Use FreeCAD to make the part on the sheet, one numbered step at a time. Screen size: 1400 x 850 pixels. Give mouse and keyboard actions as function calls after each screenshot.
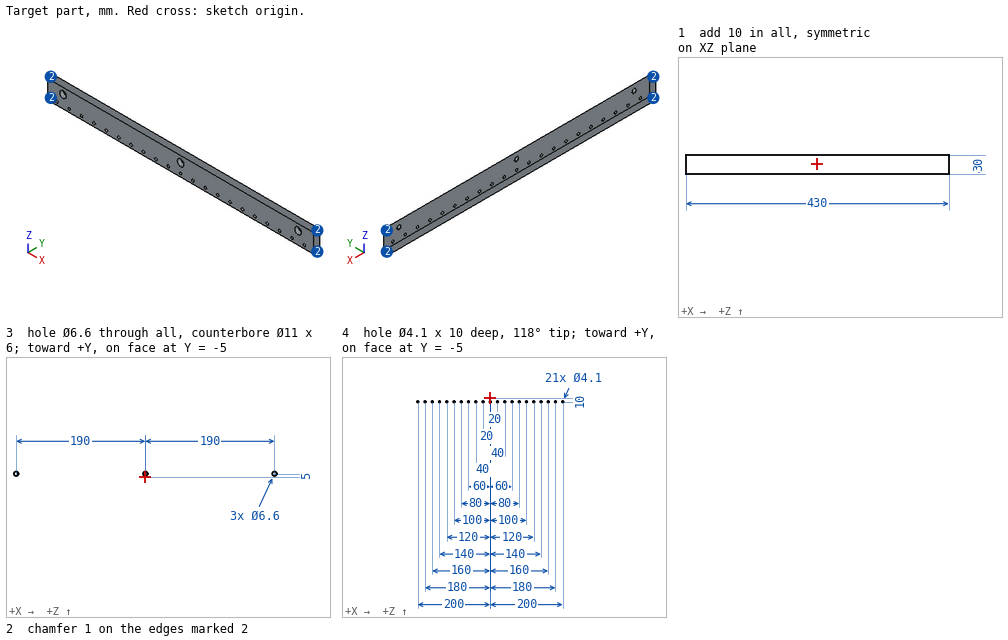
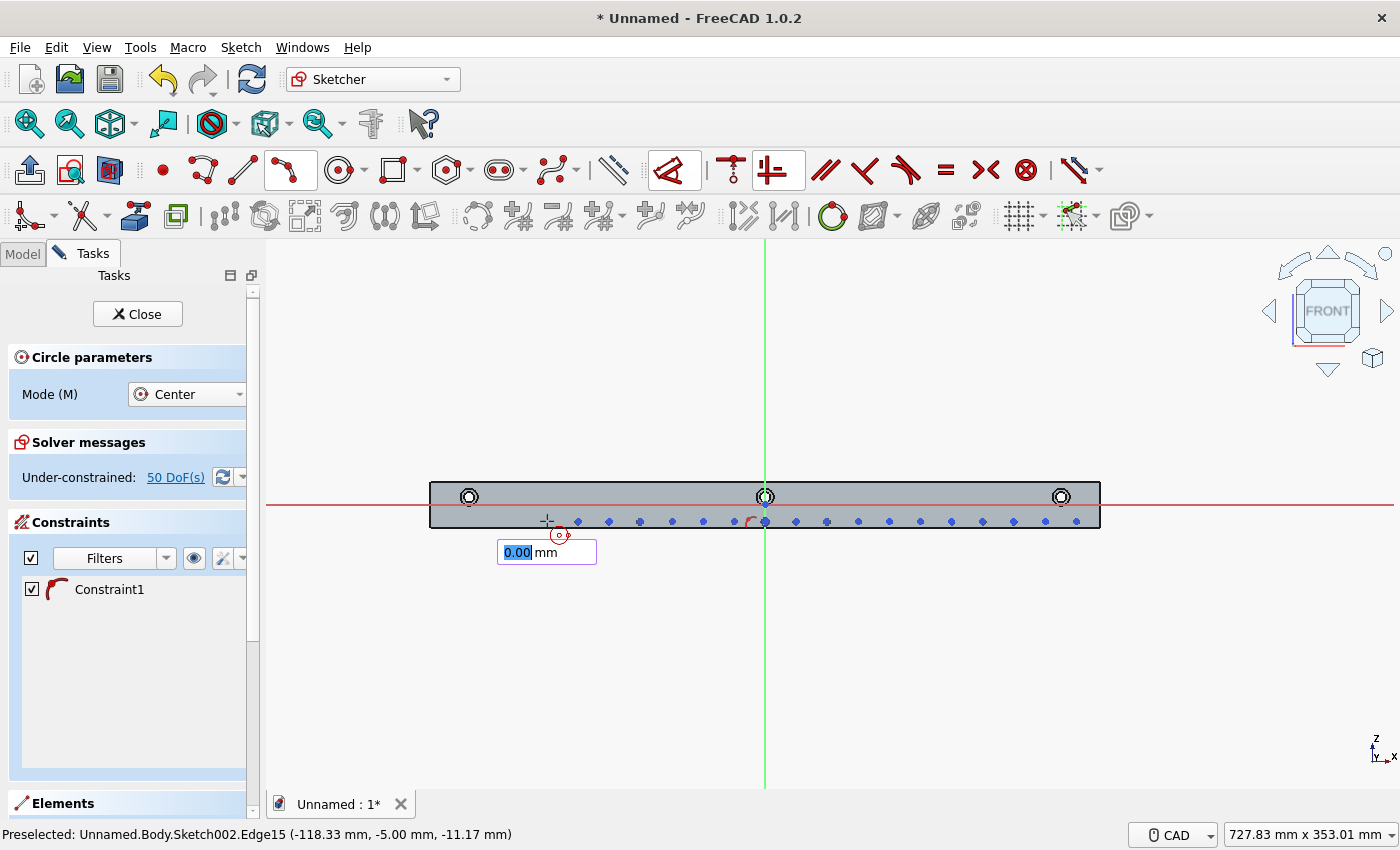
scroll(549, 523, up, 9)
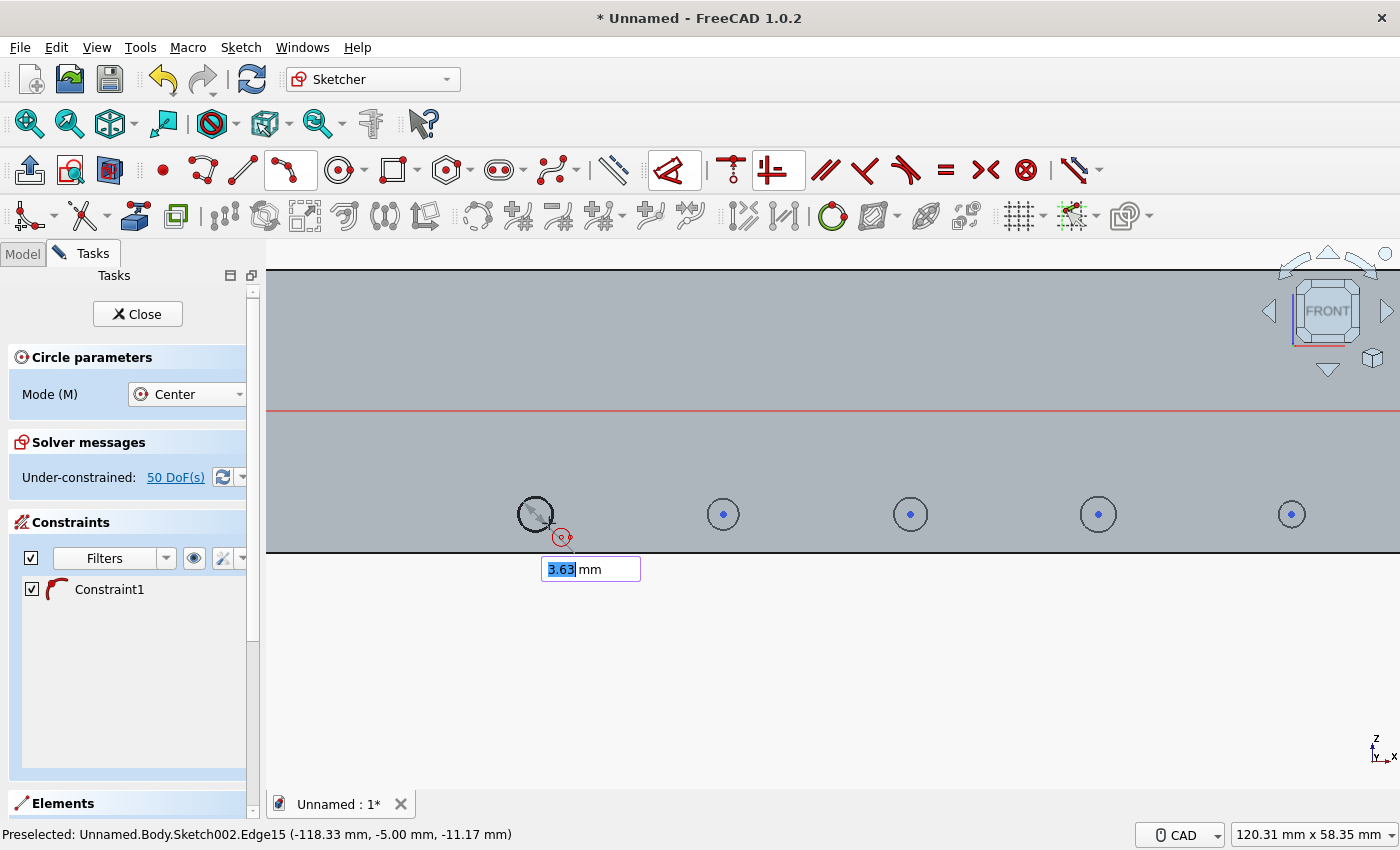
click(549, 519)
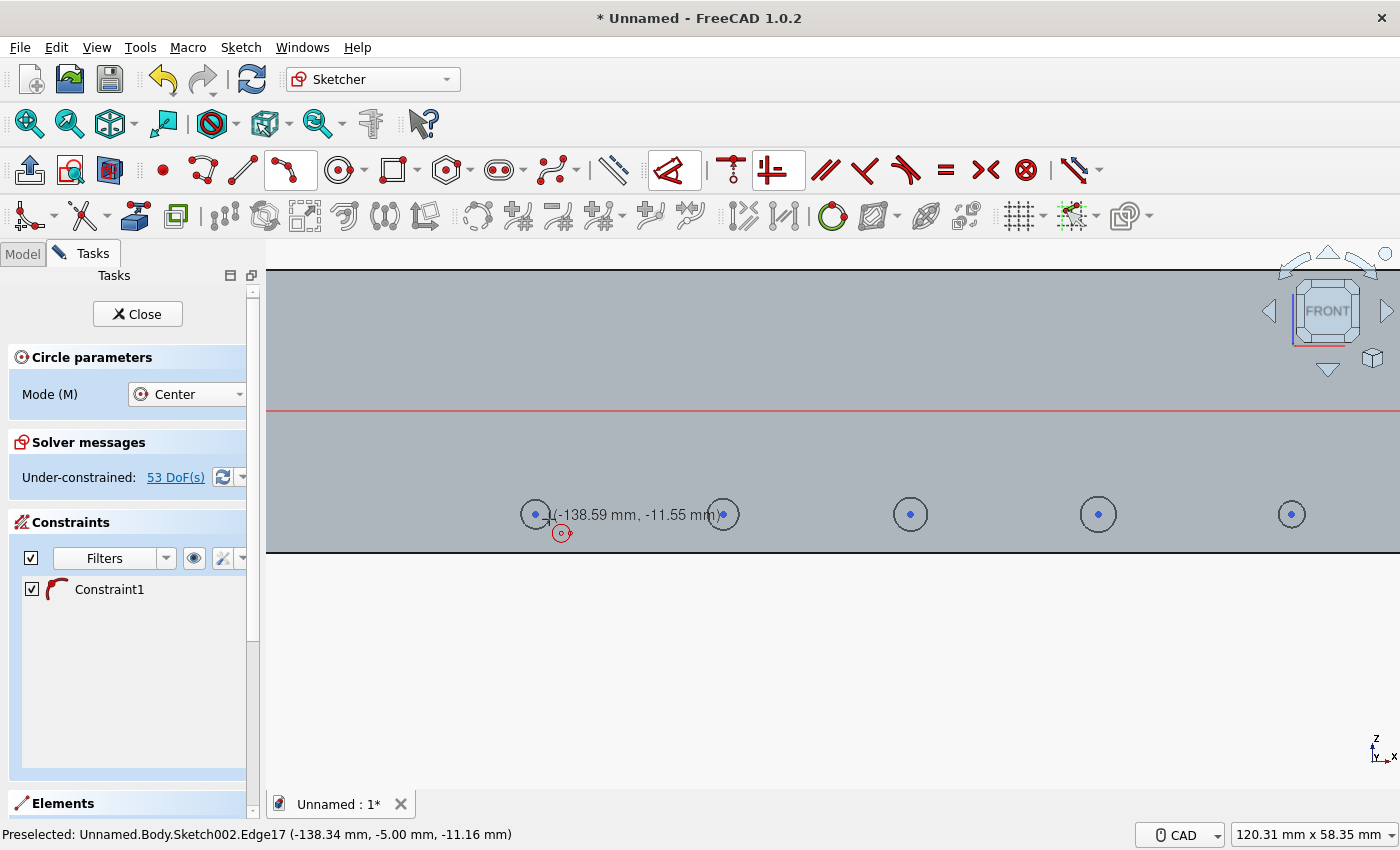
scroll(548, 523, down, 9)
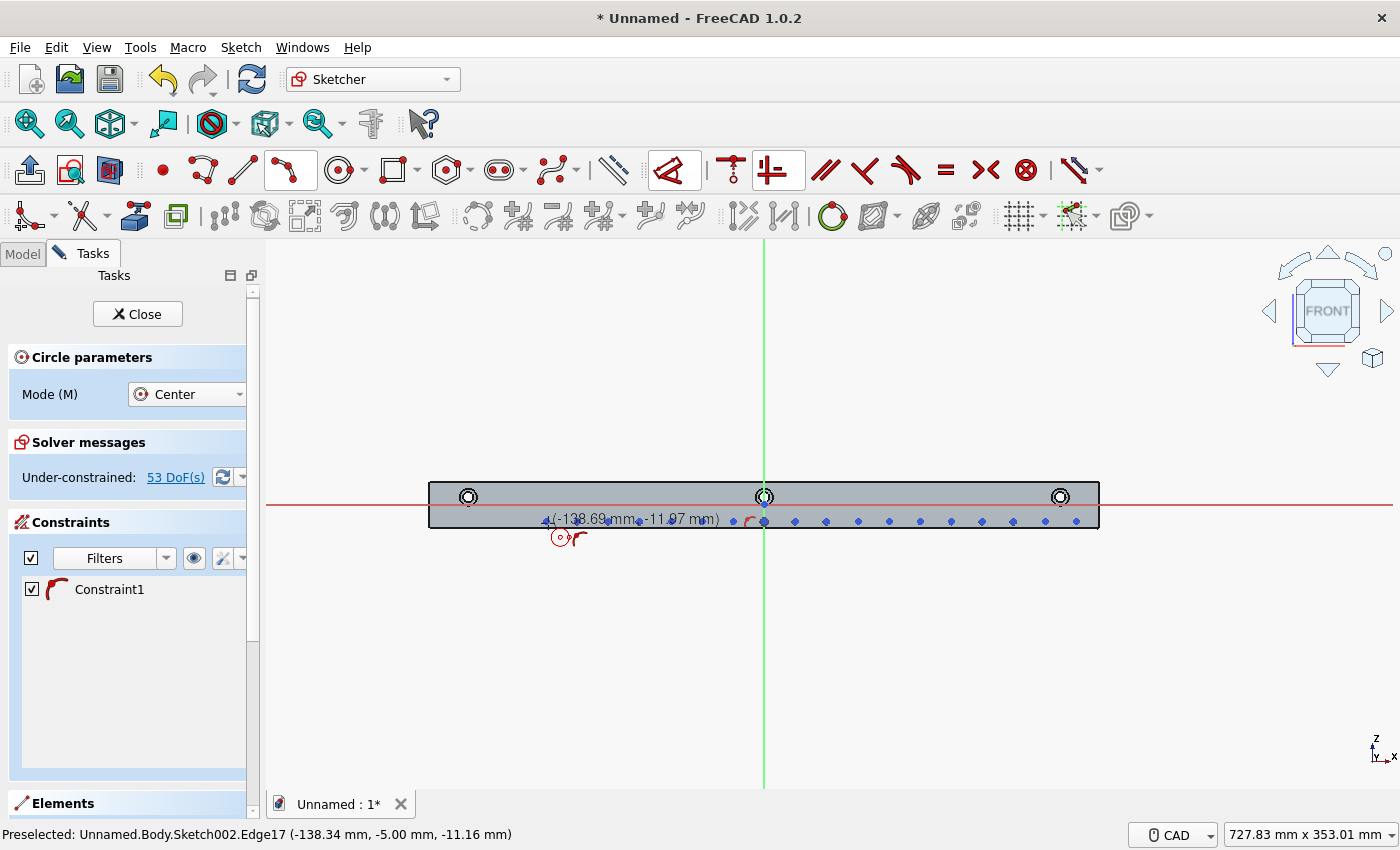
click(515, 521)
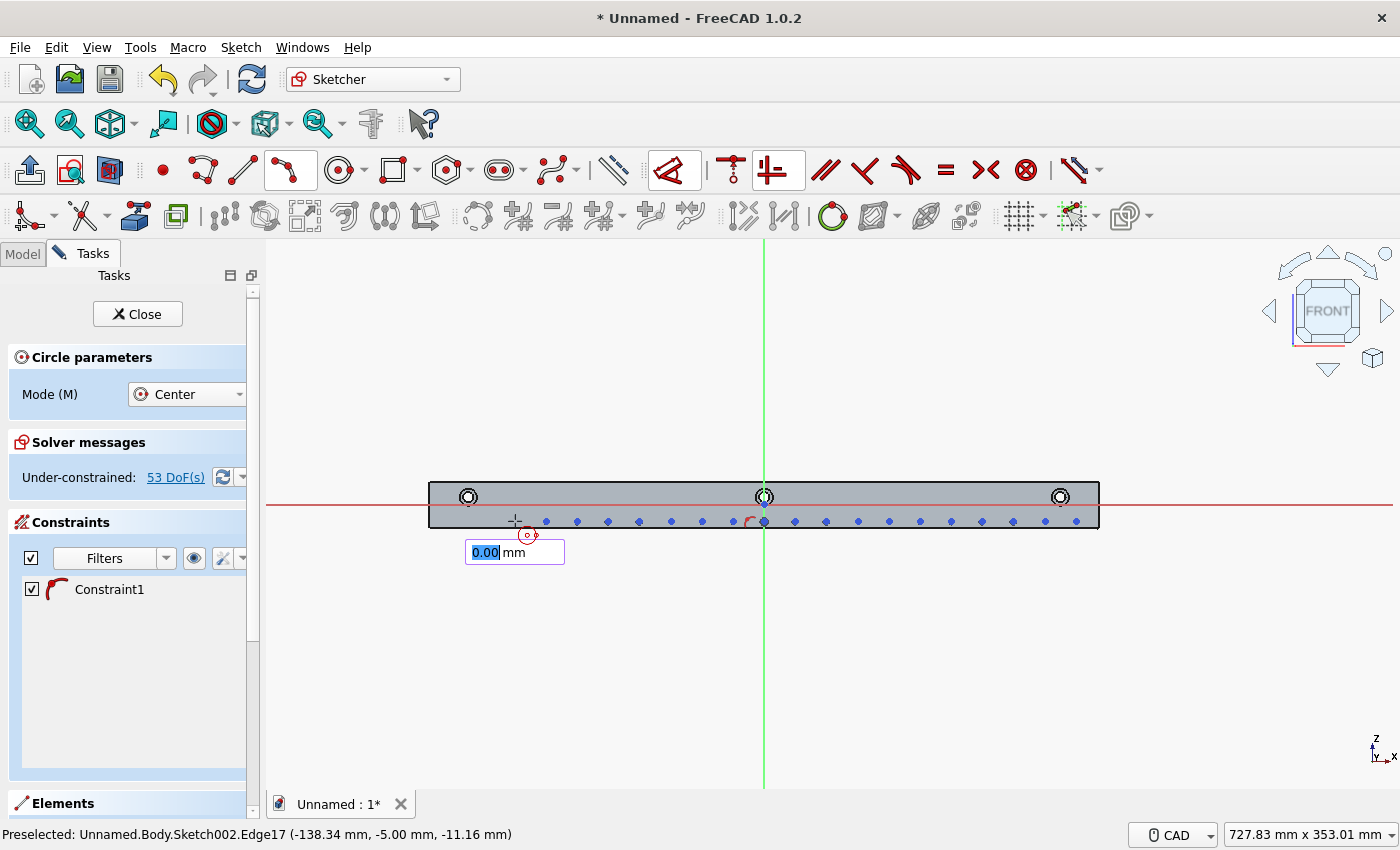
scroll(517, 523, up, 9)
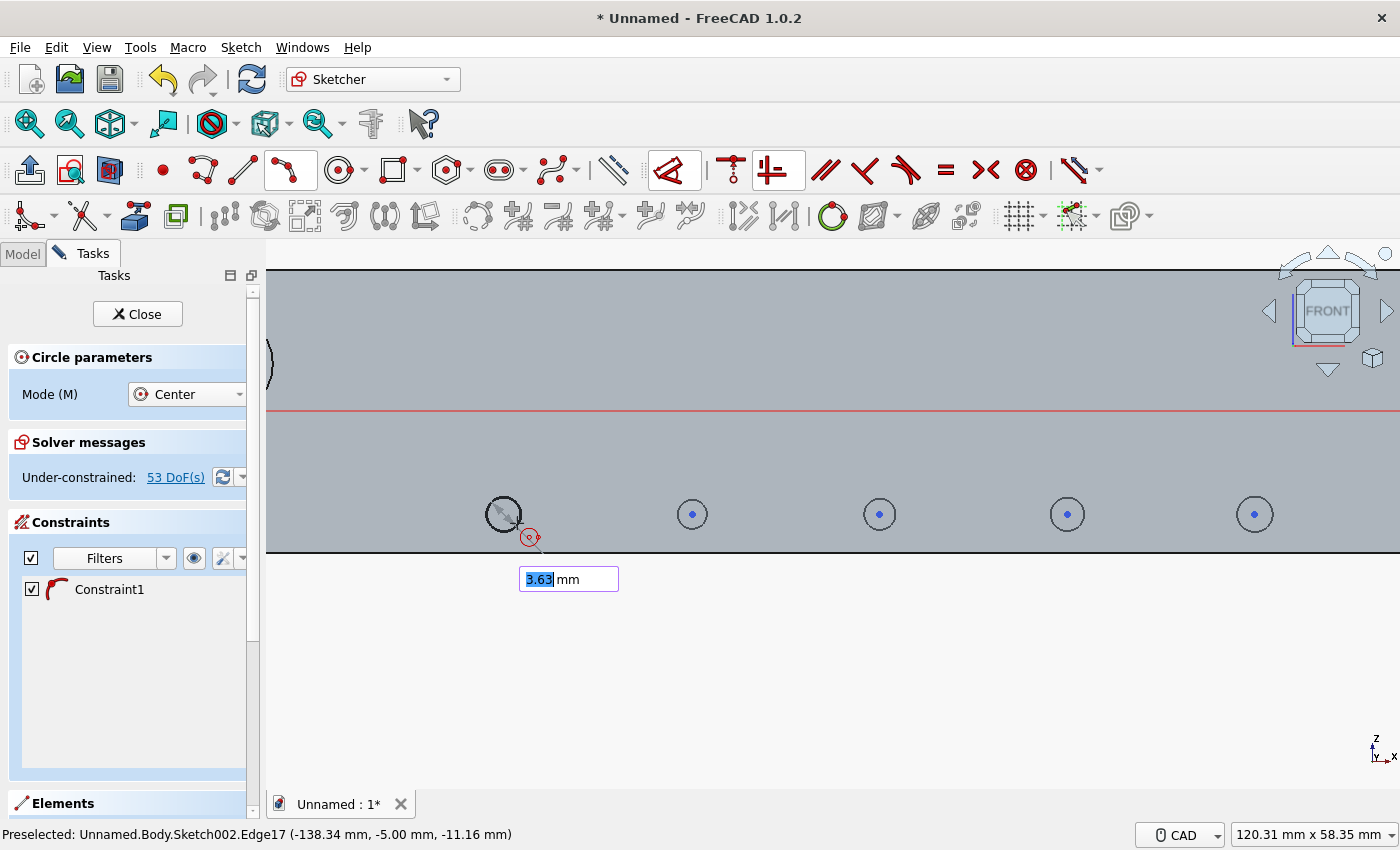
click(517, 519)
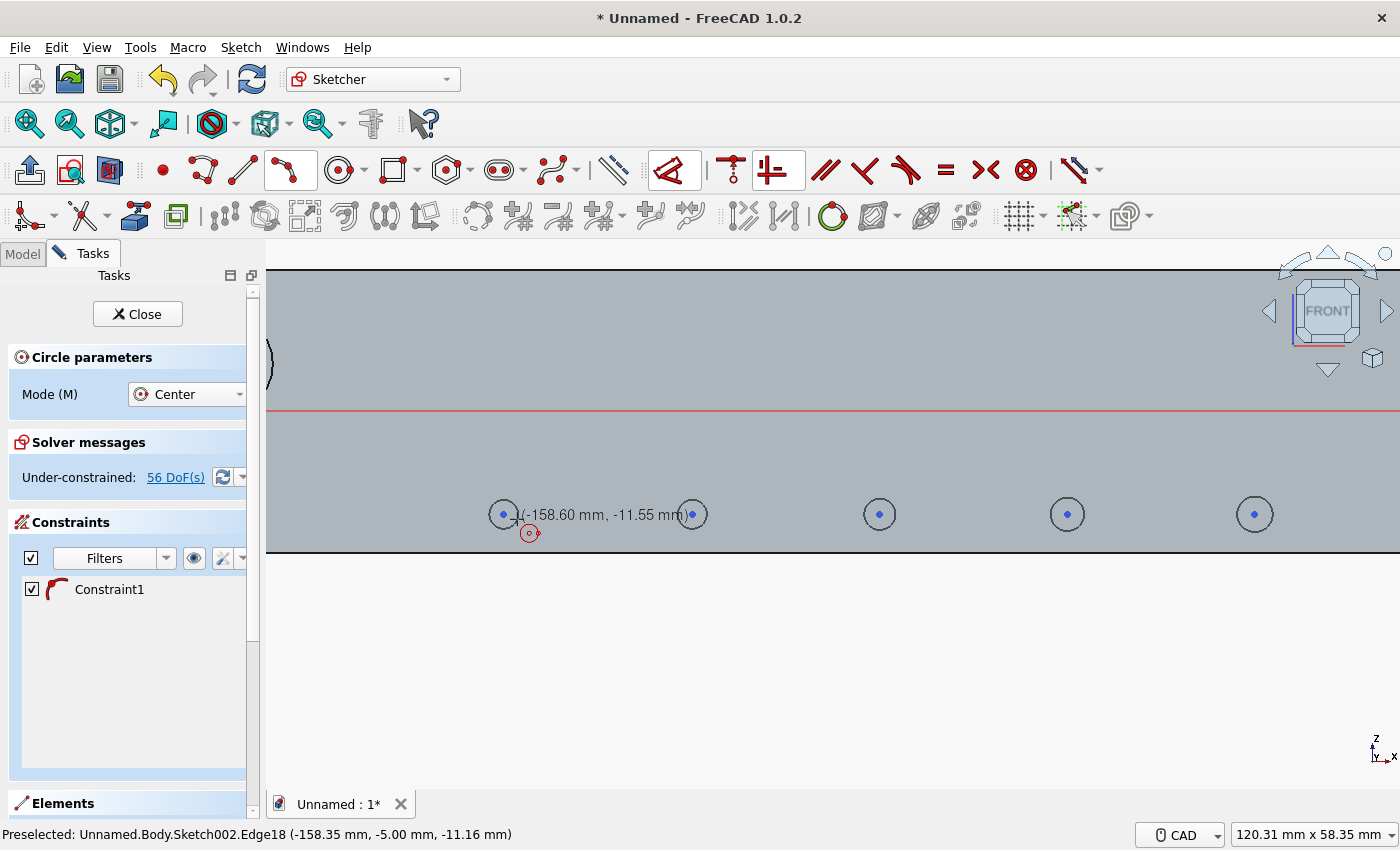
scroll(517, 523, down, 9)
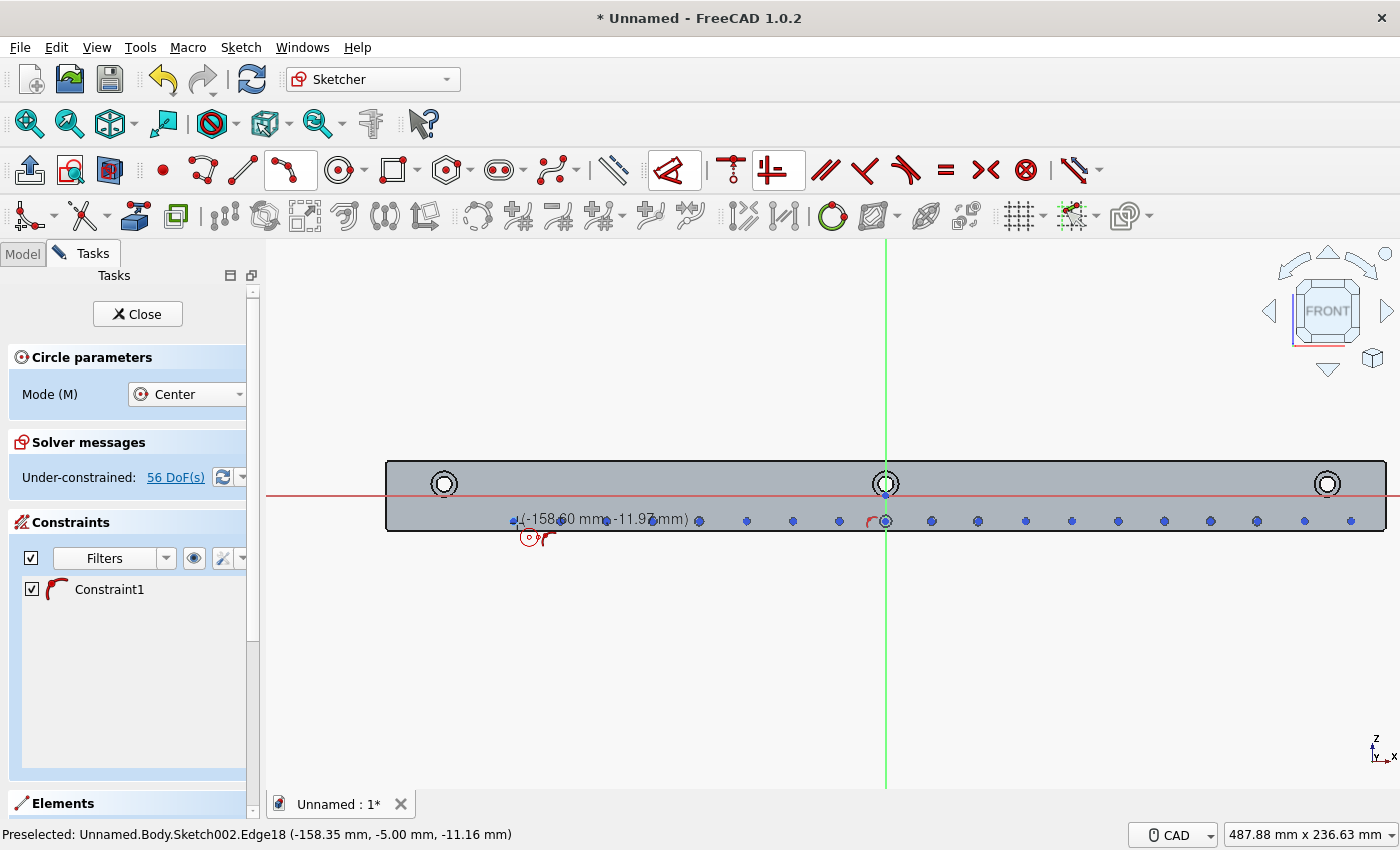
click(484, 521)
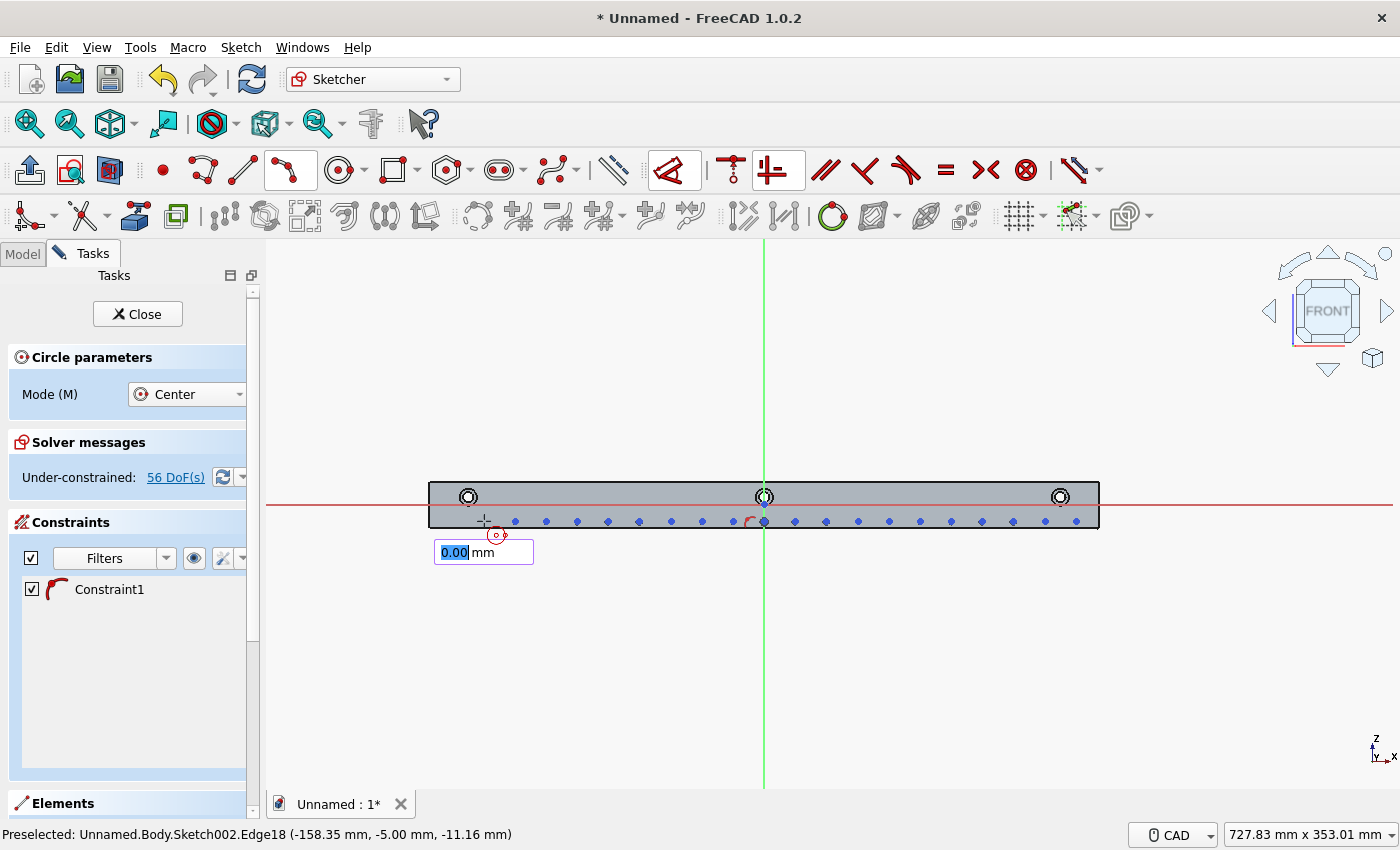
scroll(486, 523, up, 9)